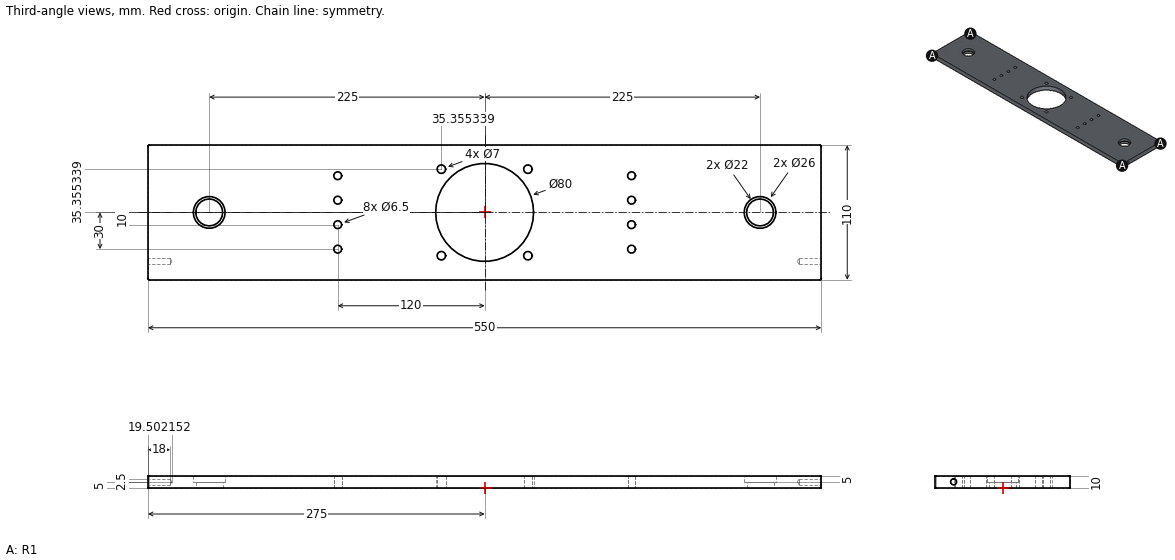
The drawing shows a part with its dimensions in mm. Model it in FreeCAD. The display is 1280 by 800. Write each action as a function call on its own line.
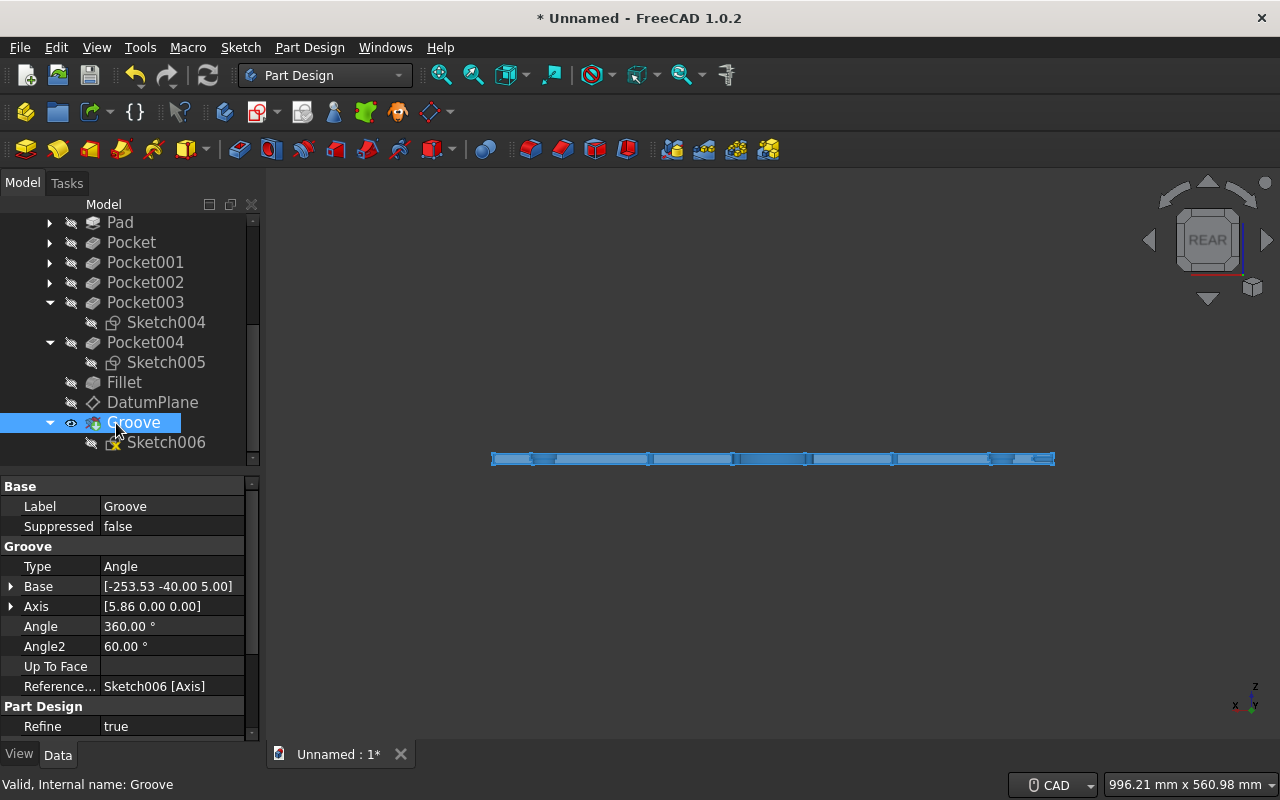
click(672, 150)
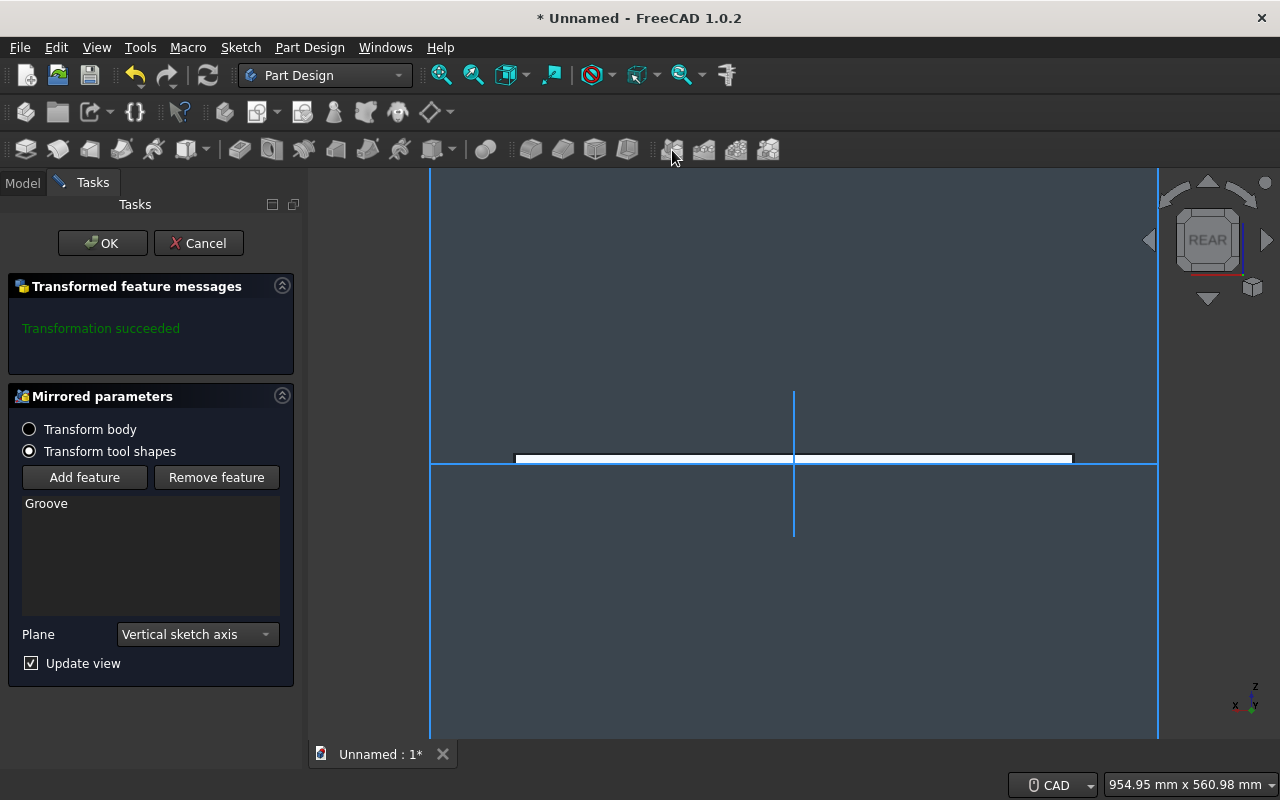
click(198, 634)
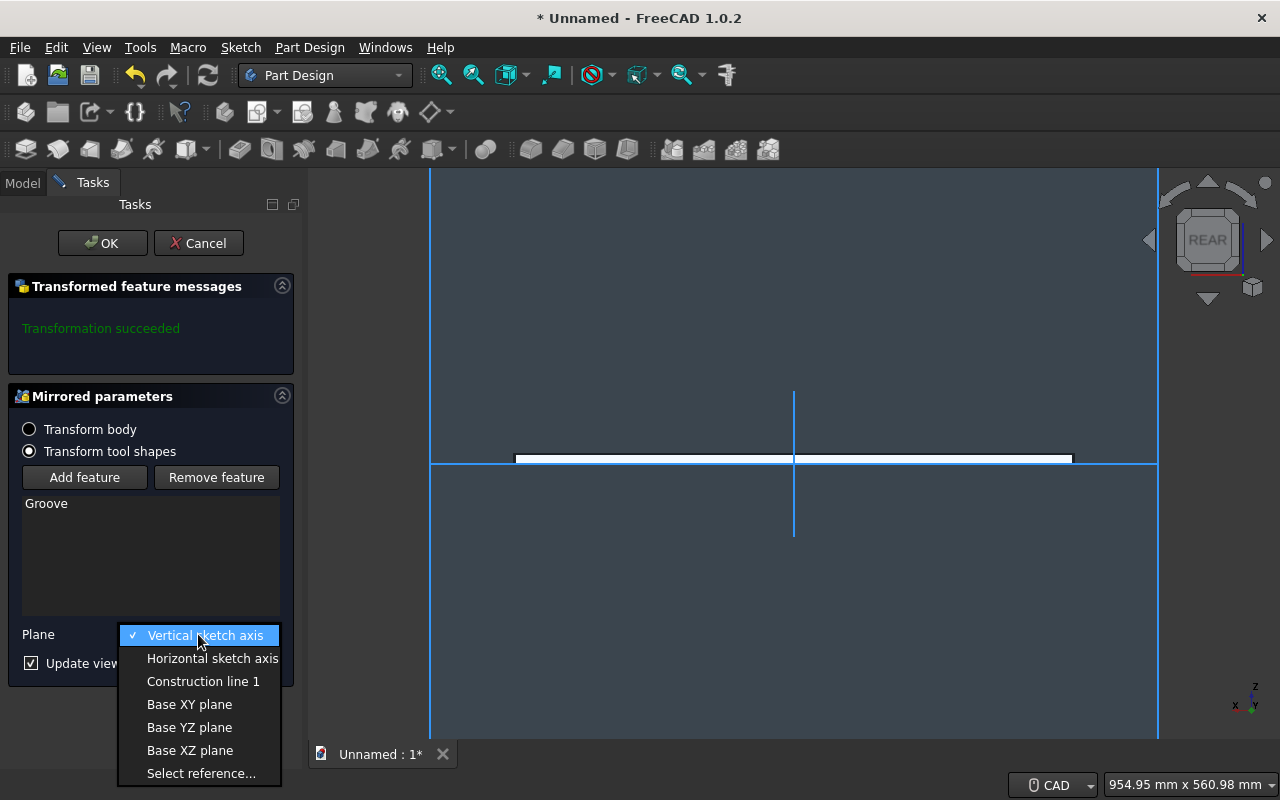
click(198, 728)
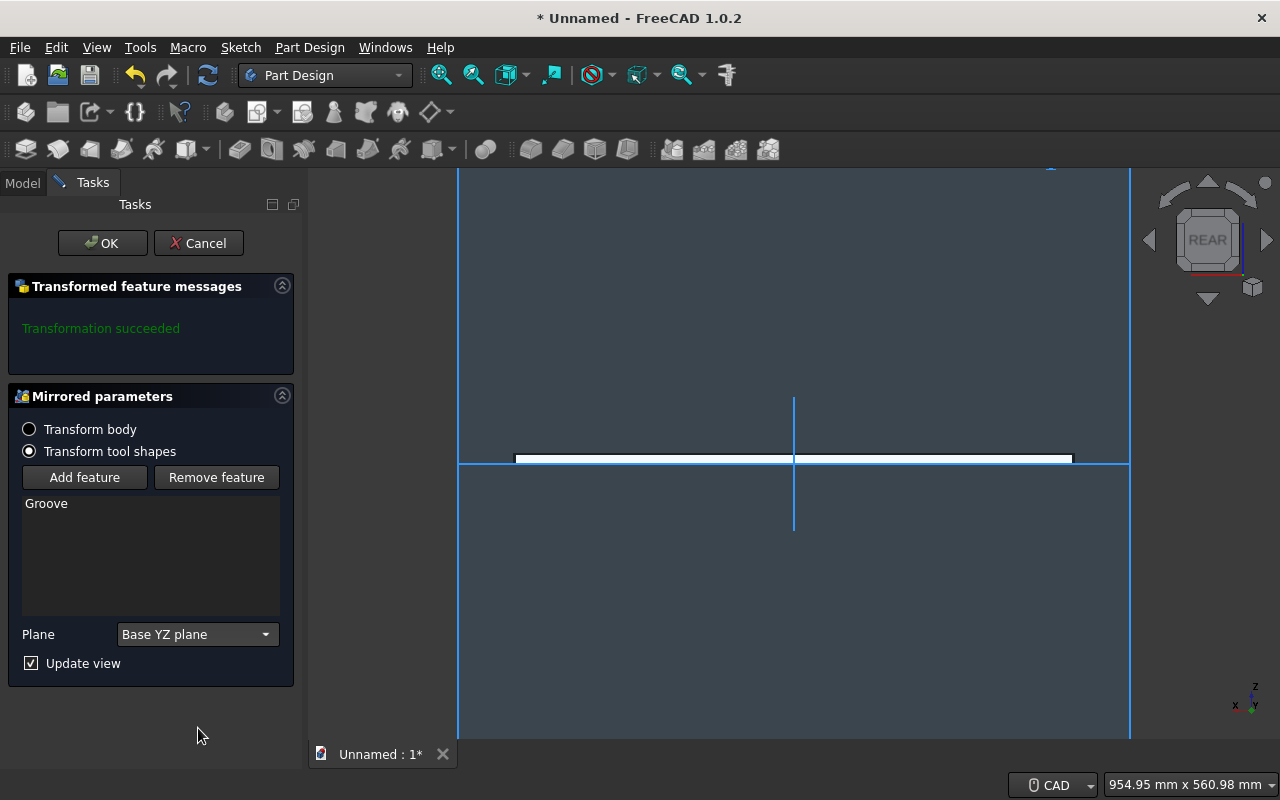
click(103, 243)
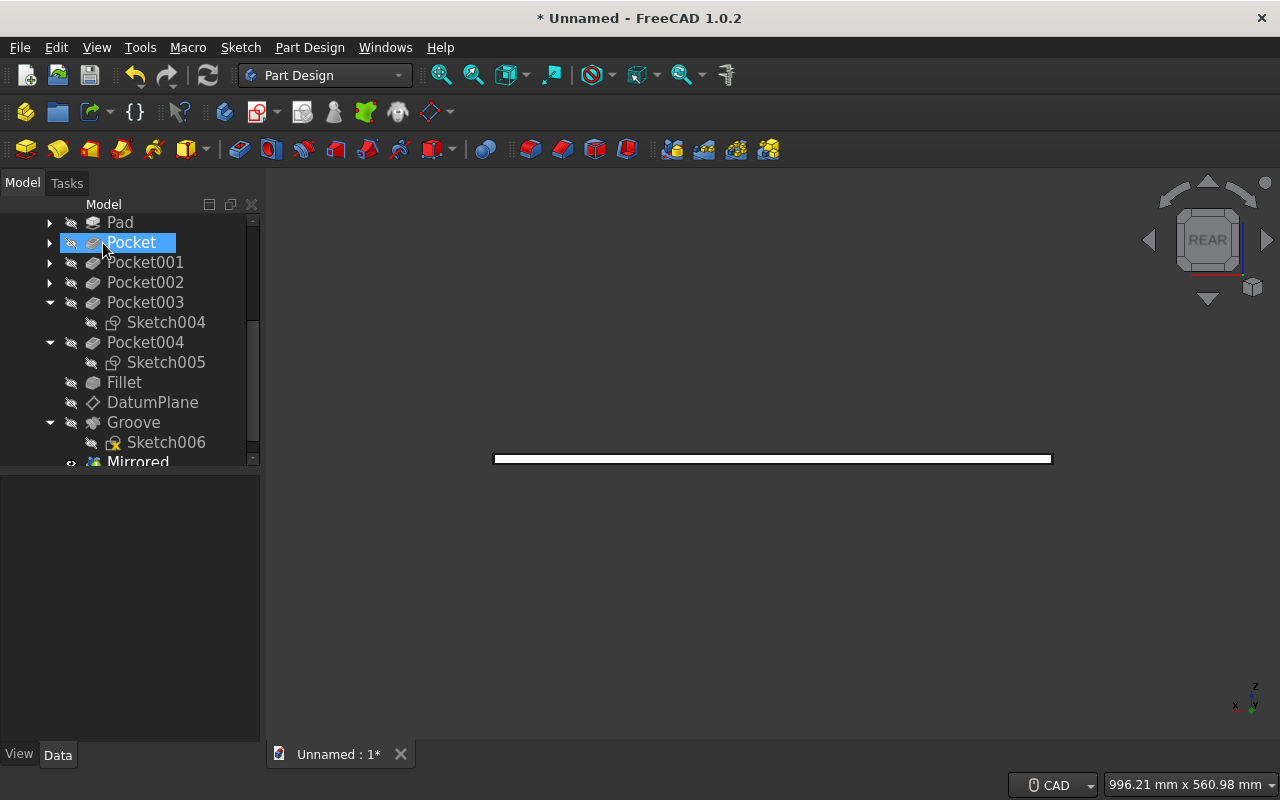
key(0)